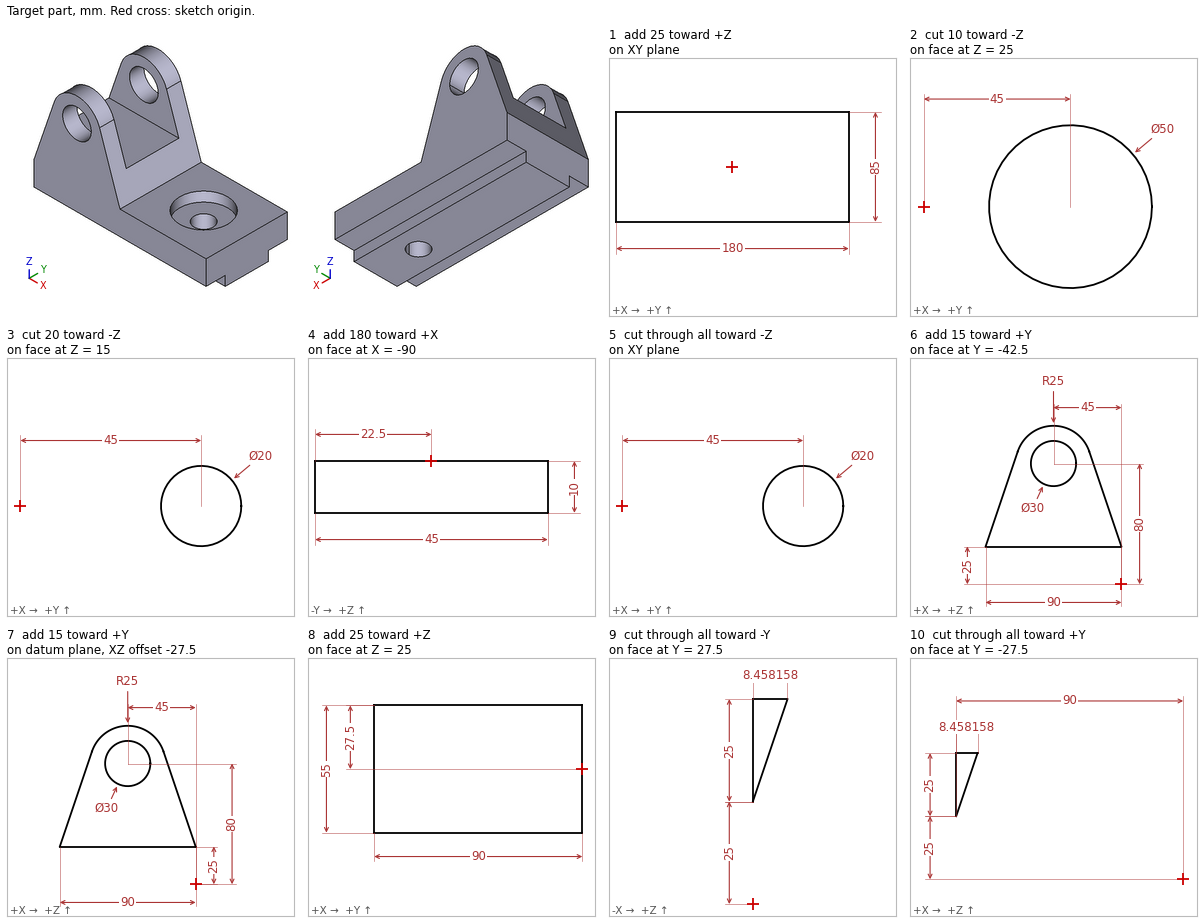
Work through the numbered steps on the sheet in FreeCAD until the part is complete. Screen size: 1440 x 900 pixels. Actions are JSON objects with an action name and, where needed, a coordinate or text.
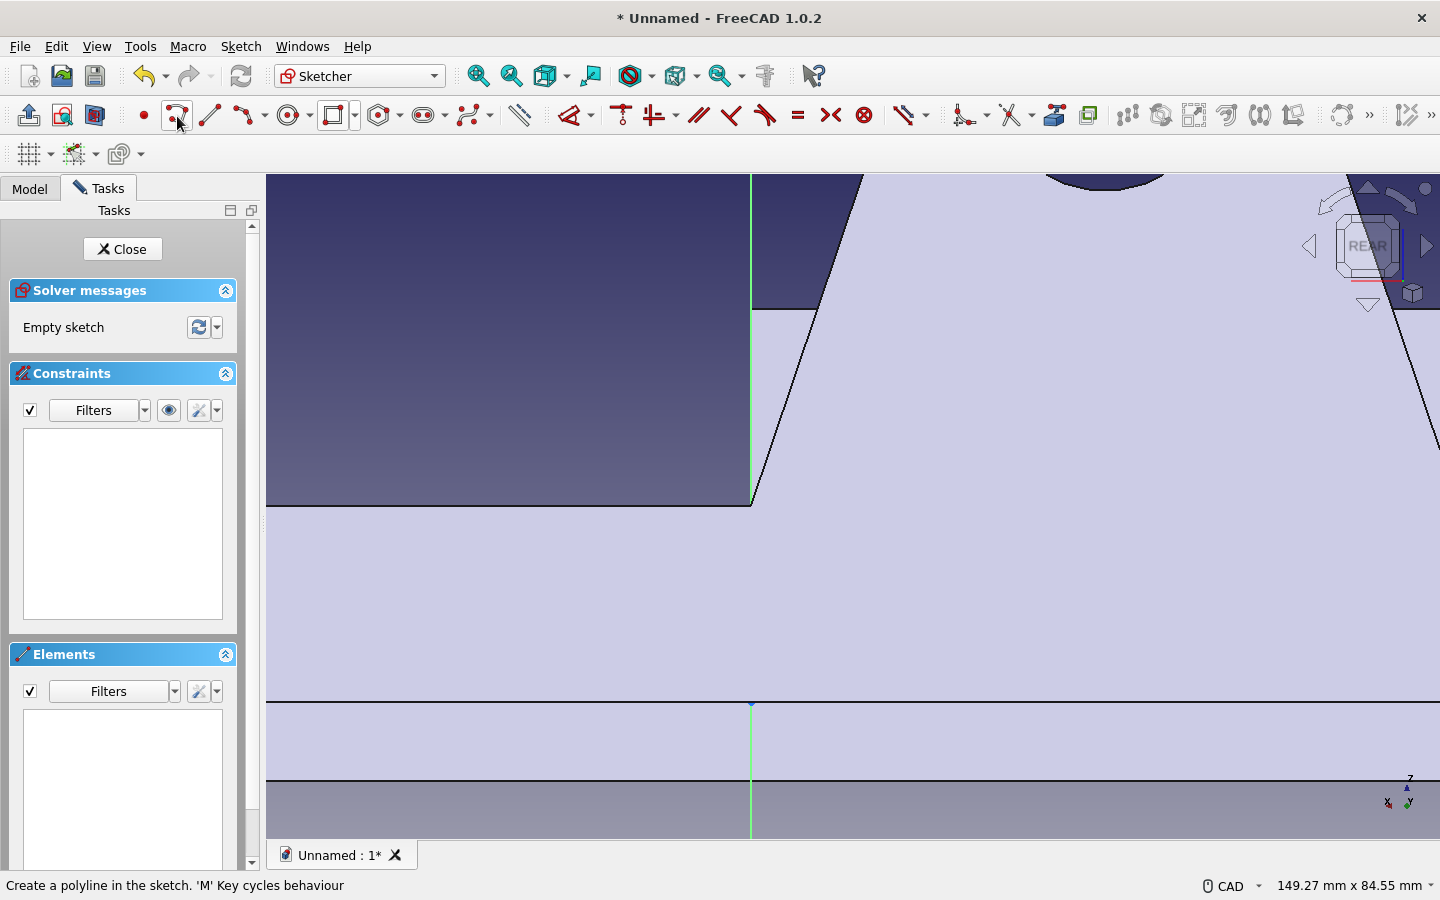
{"action": "left_click", "coordinate": [751, 506]}
{"action": "left_click", "coordinate": [818, 309]}
{"action": "left_click", "coordinate": [760, 309]}
{"action": "left_click", "coordinate": [751, 507]}
{"action": "key", "text": "Escape"}
{"action": "key", "text": "Escape"}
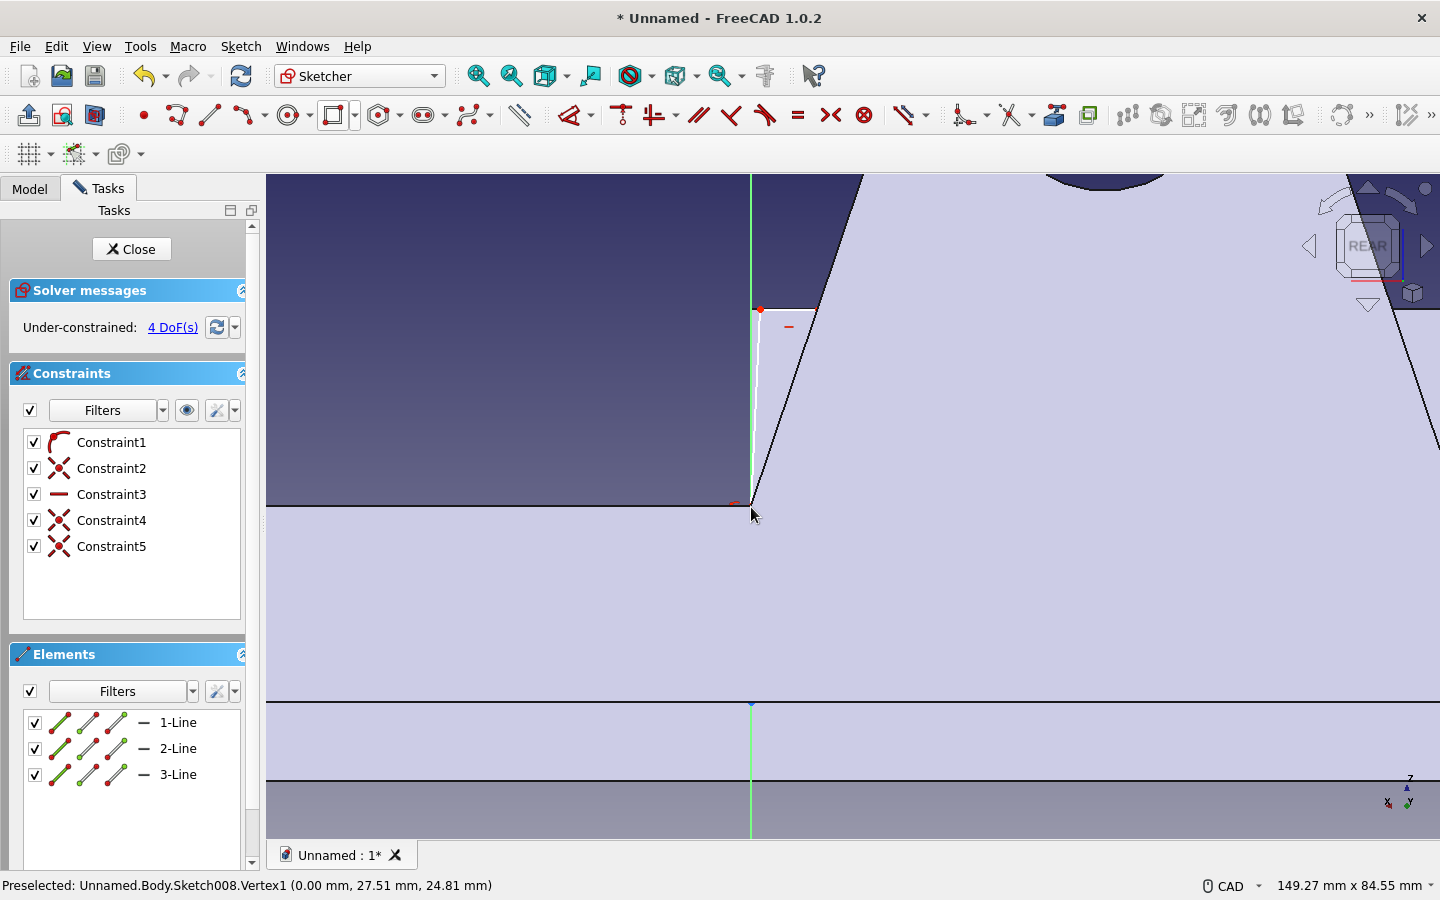
{"action": "left_click", "coordinate": [754, 448]}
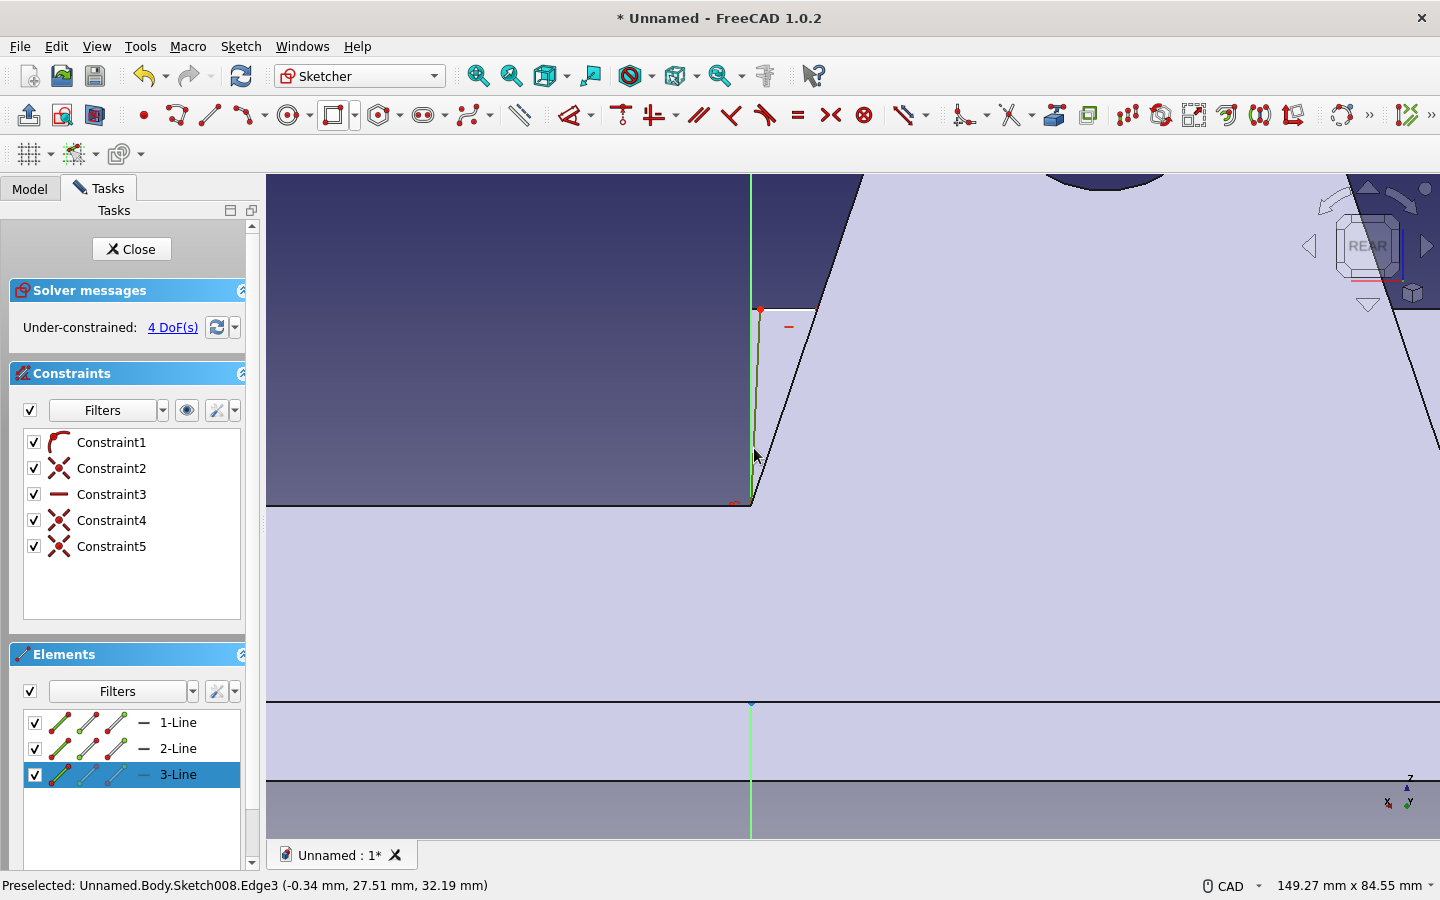
{"action": "left_click", "coordinate": [676, 116]}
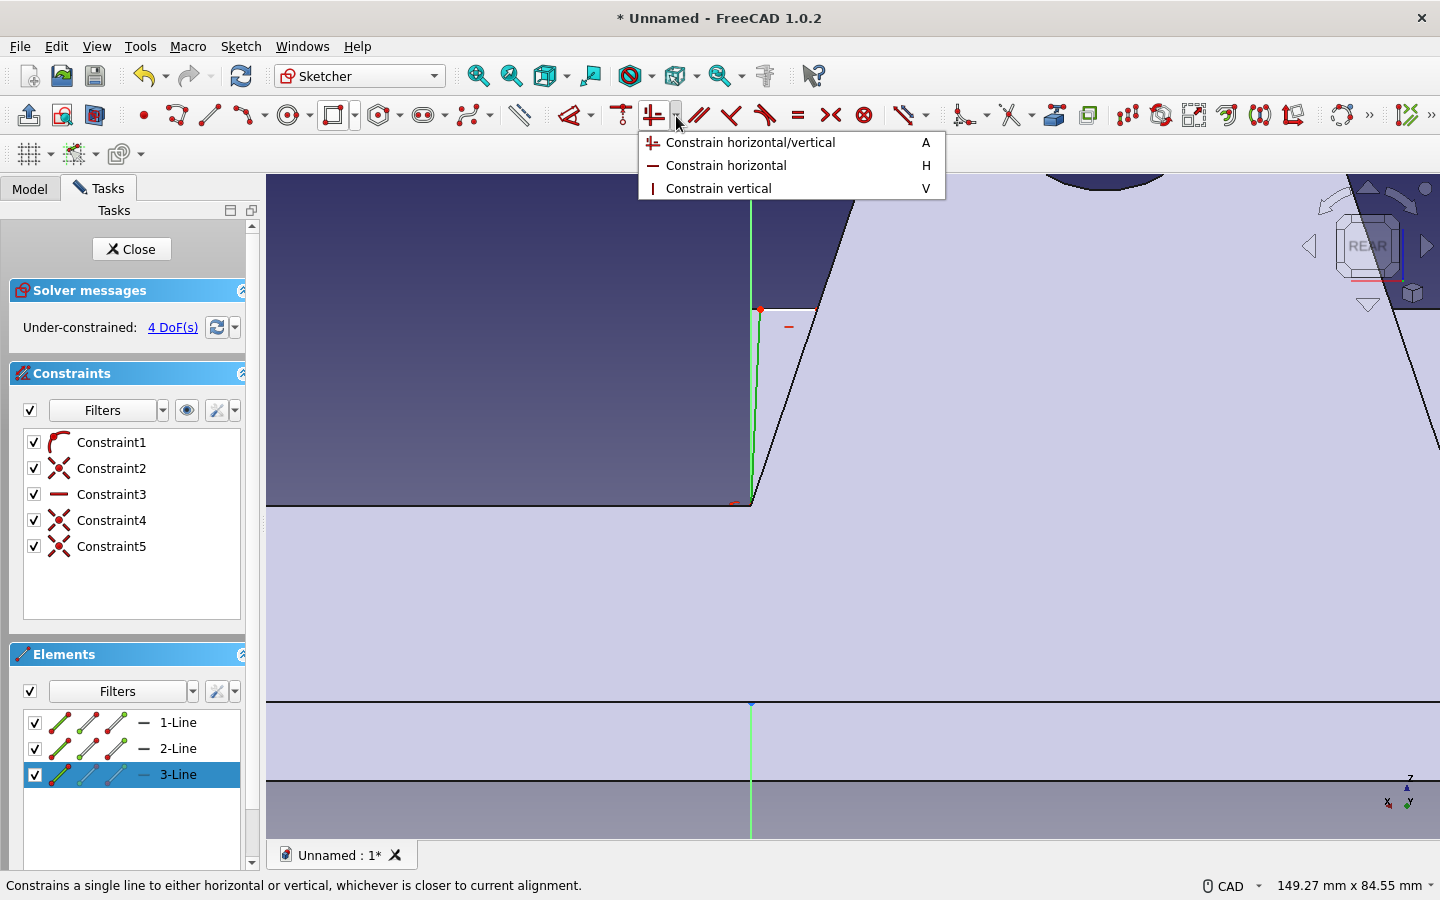
{"action": "left_click", "coordinate": [792, 188]}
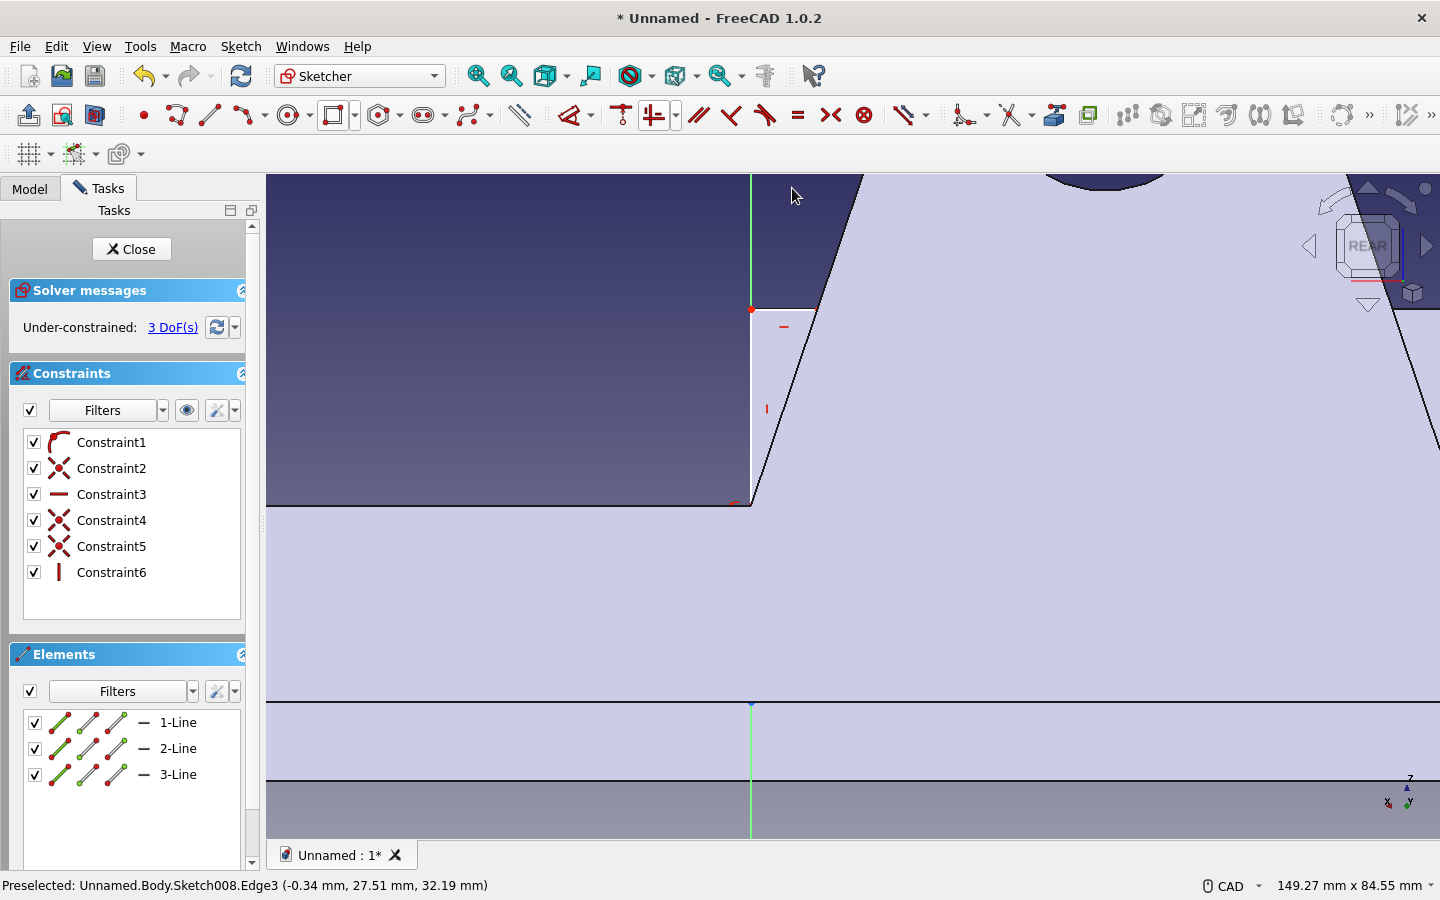
{"action": "left_click", "coordinate": [568, 116]}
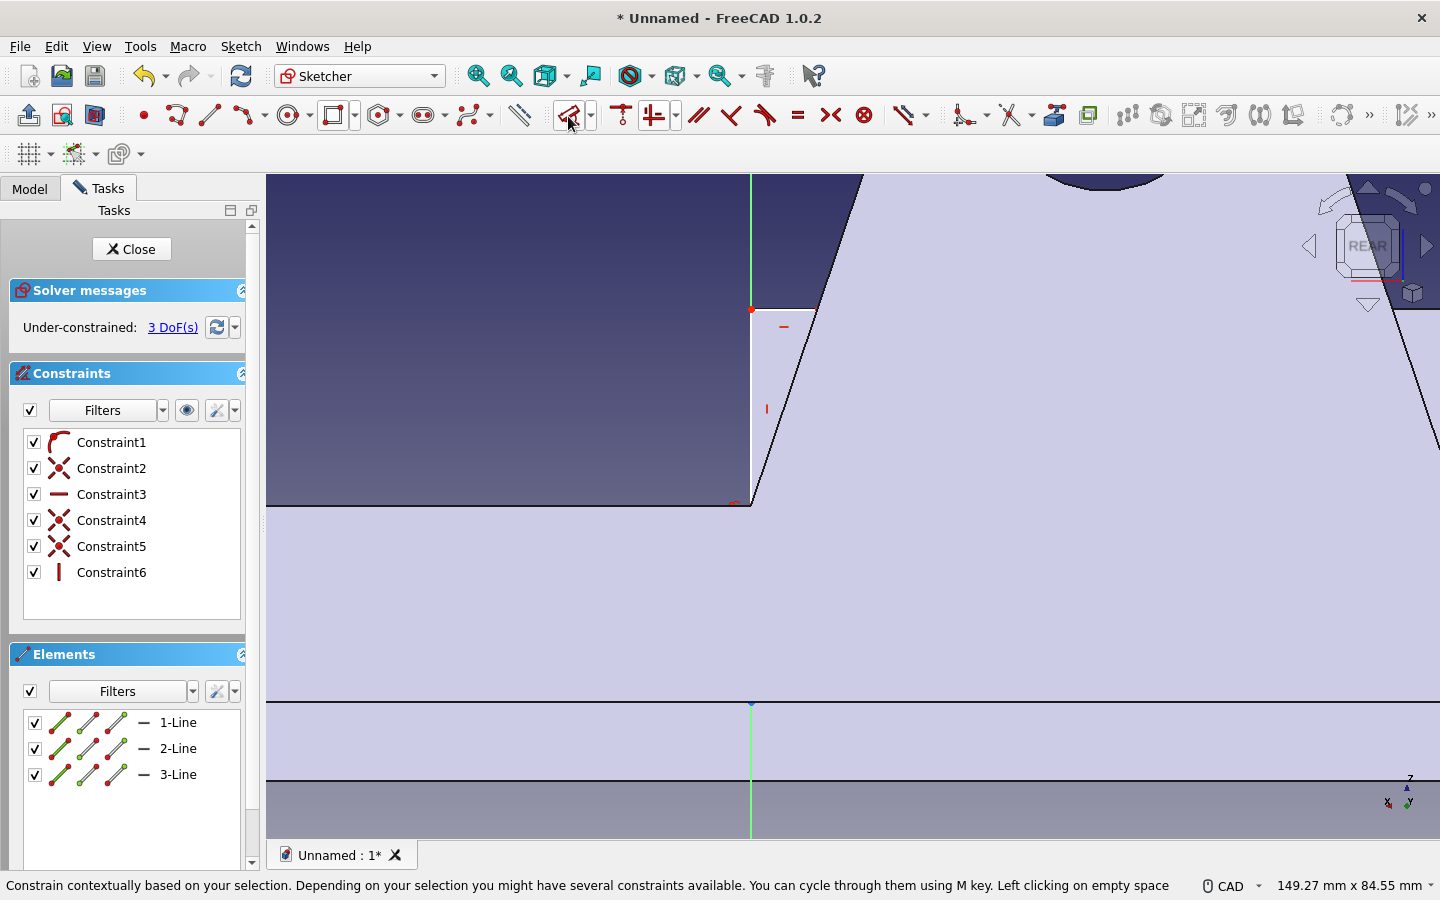
{"action": "left_click", "coordinate": [751, 369]}
{"action": "left_click", "coordinate": [717, 408]}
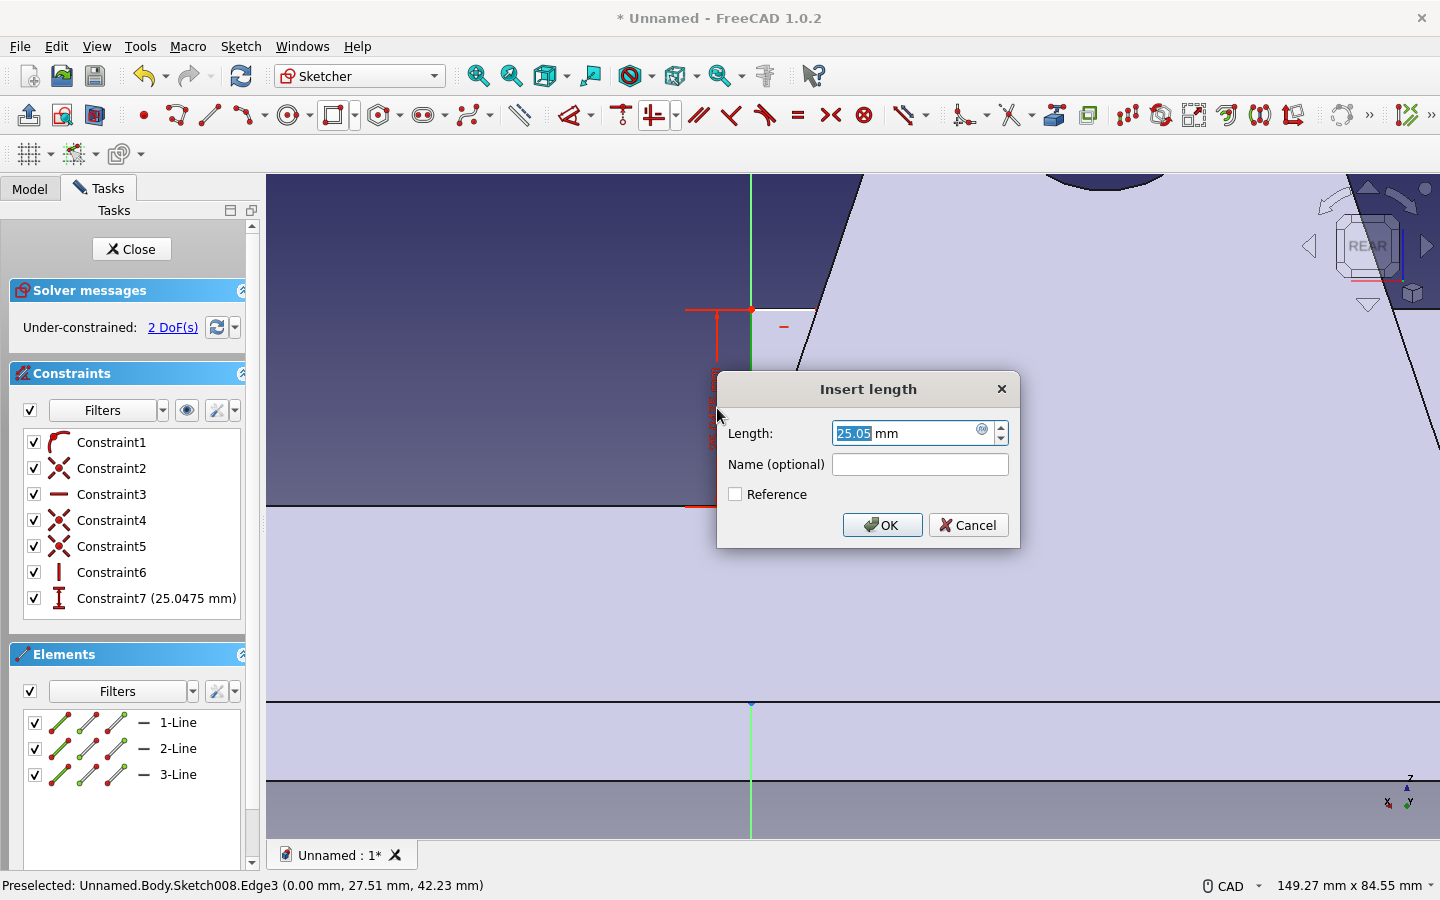
{"action": "type", "text": "25"}
{"action": "key", "text": "Return"}